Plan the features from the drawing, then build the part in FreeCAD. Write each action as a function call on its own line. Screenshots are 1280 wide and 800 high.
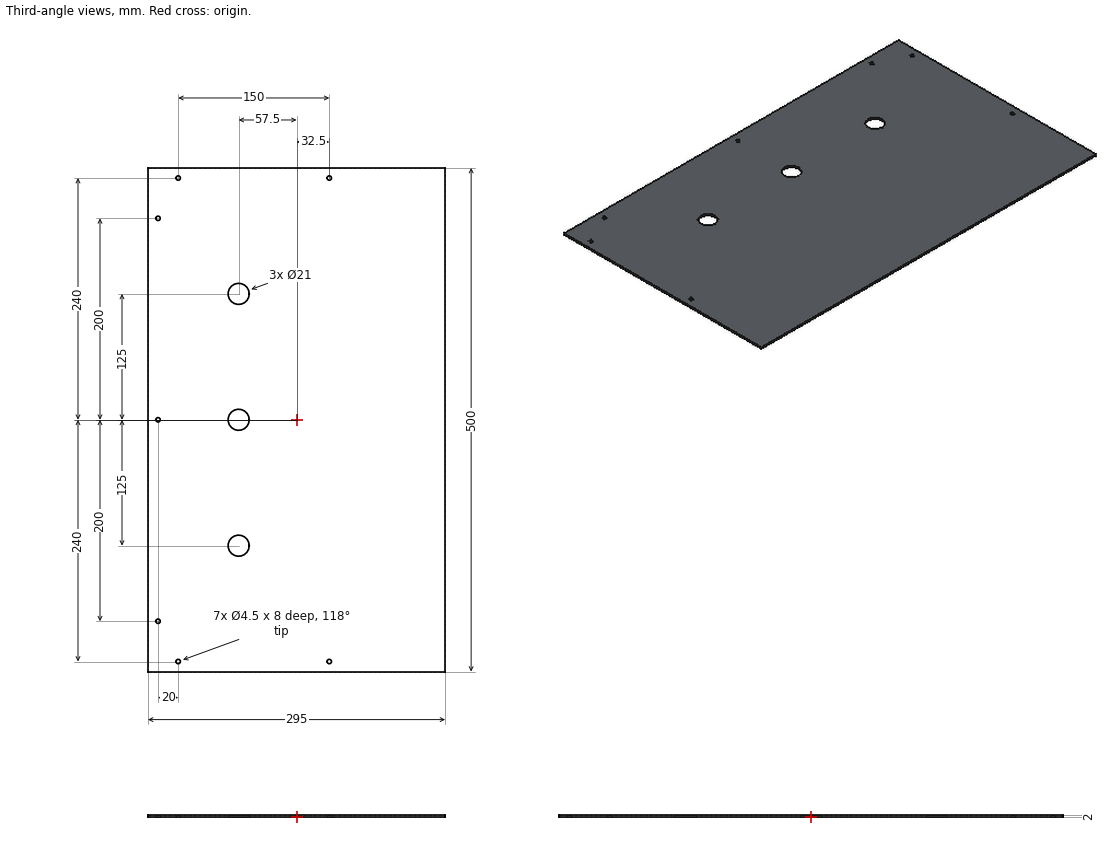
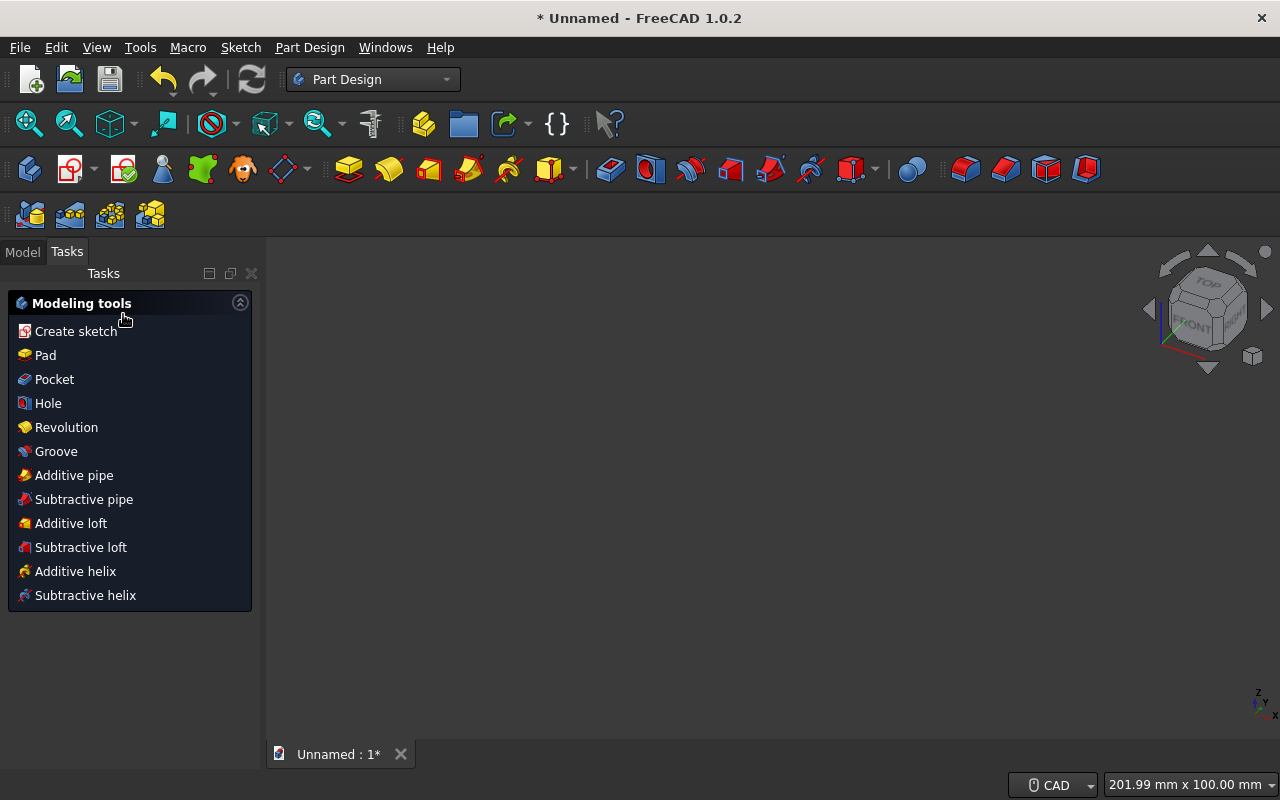
click(350, 170)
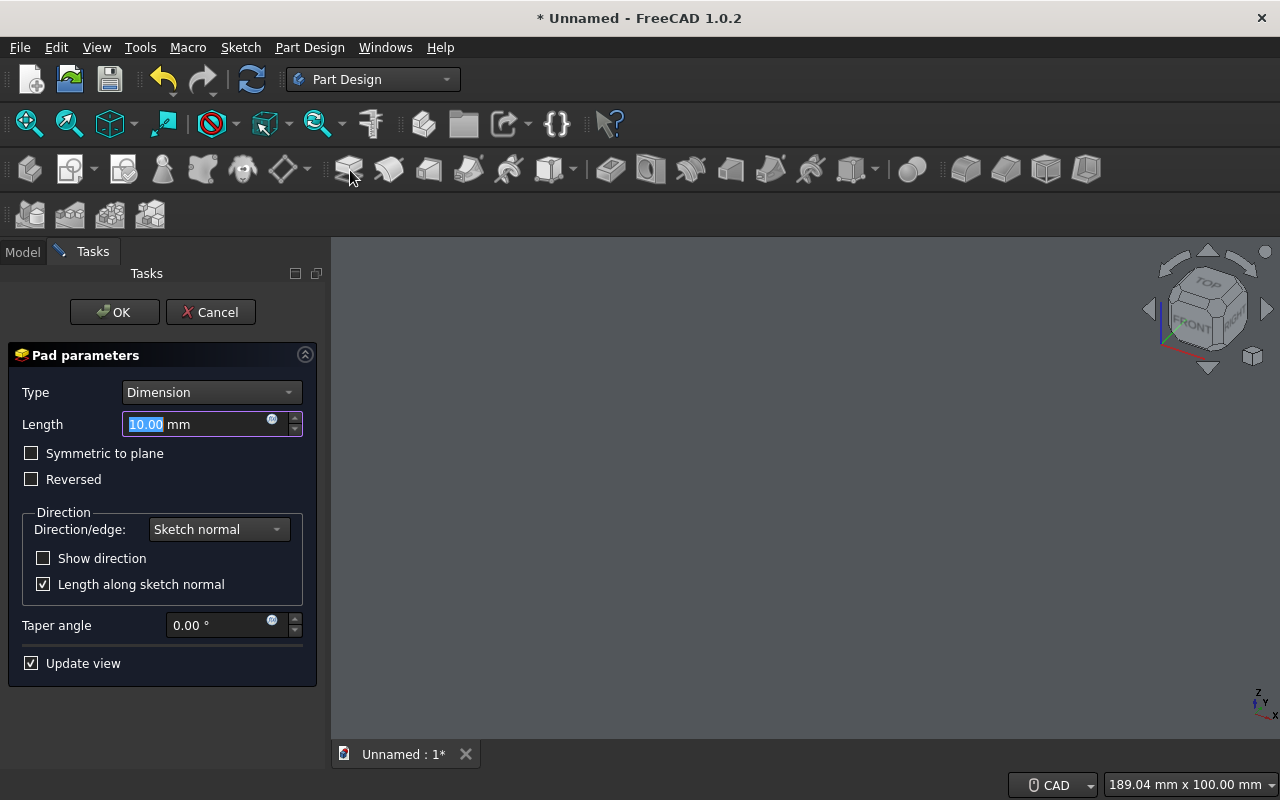
text(2)
key(Tab)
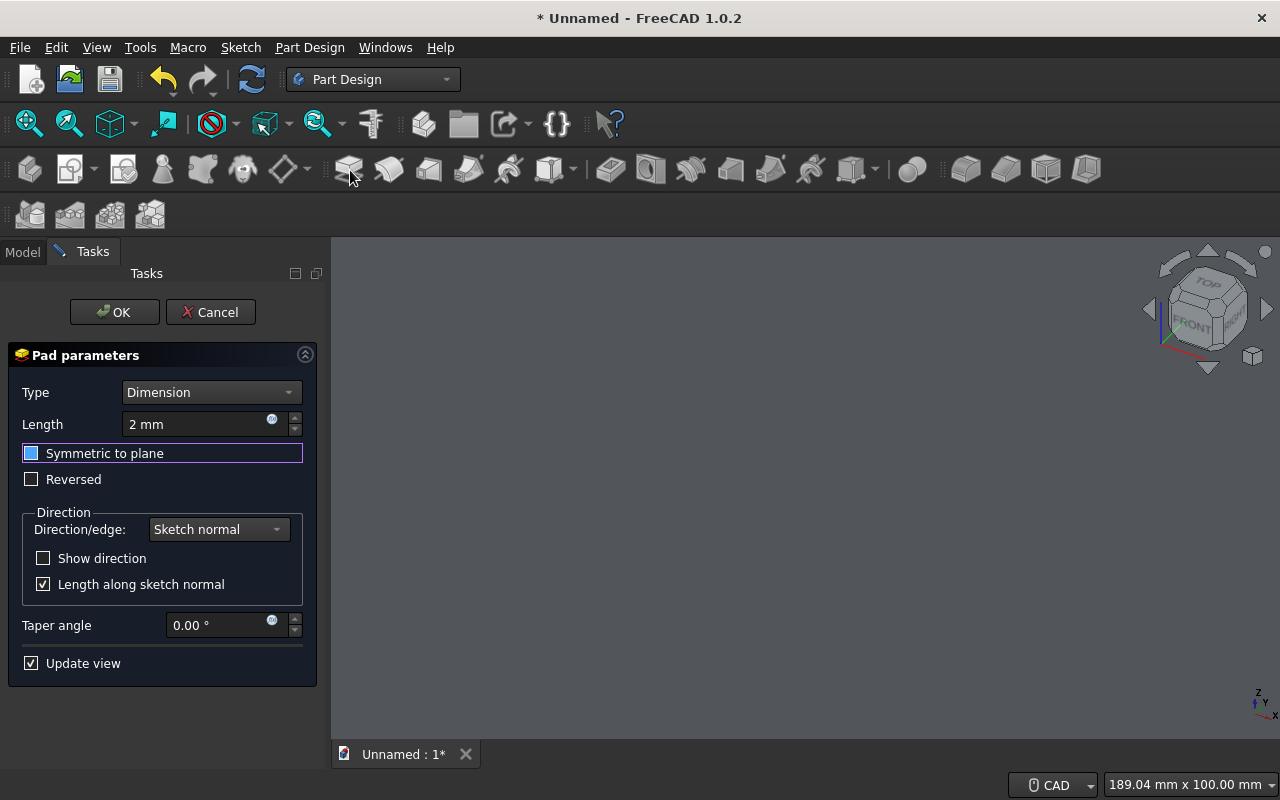
click(115, 312)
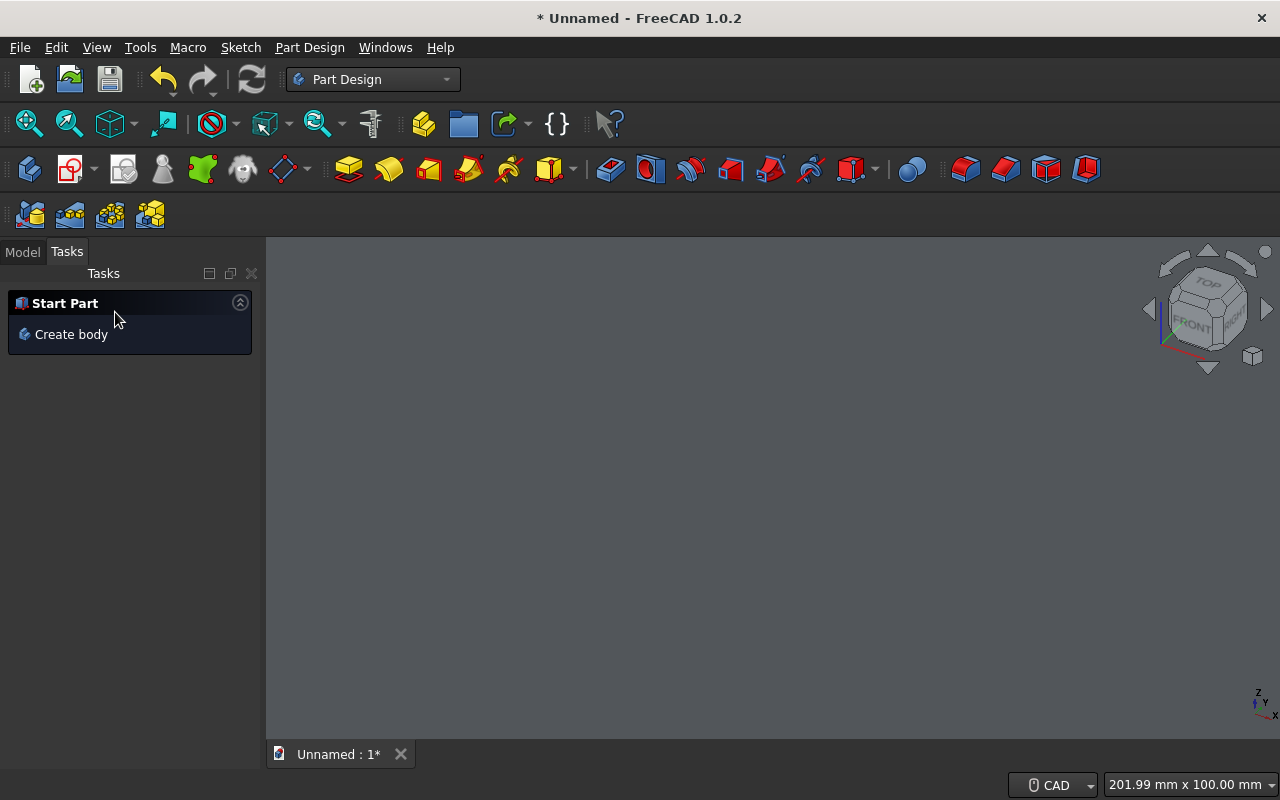
click(30, 124)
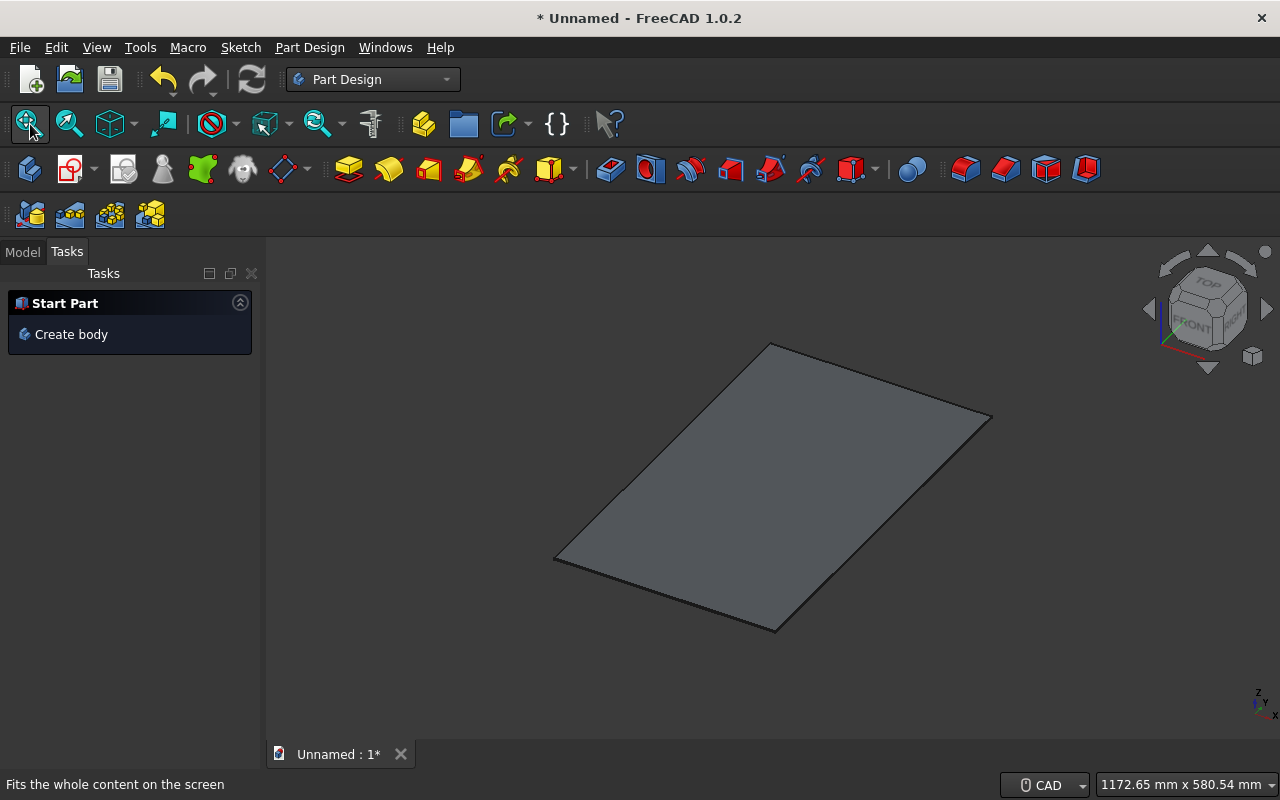
click(804, 456)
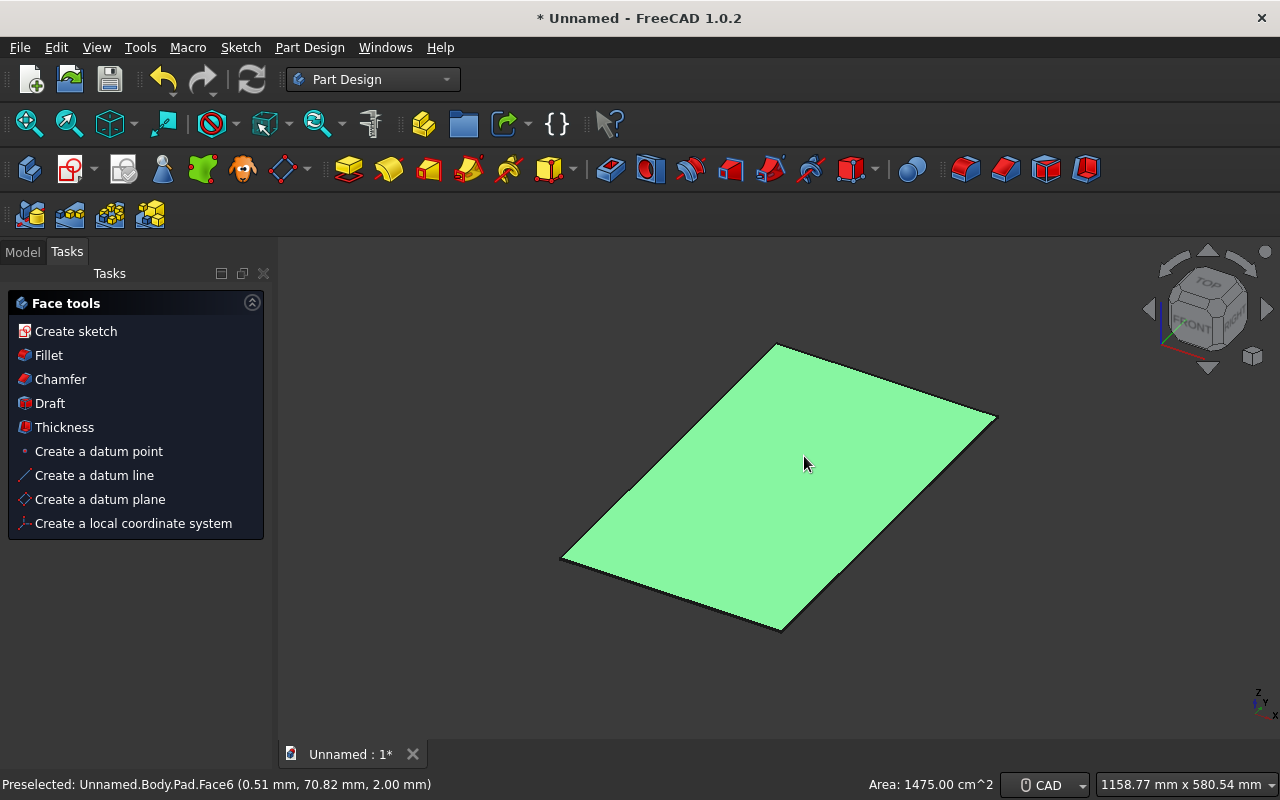
click(70, 170)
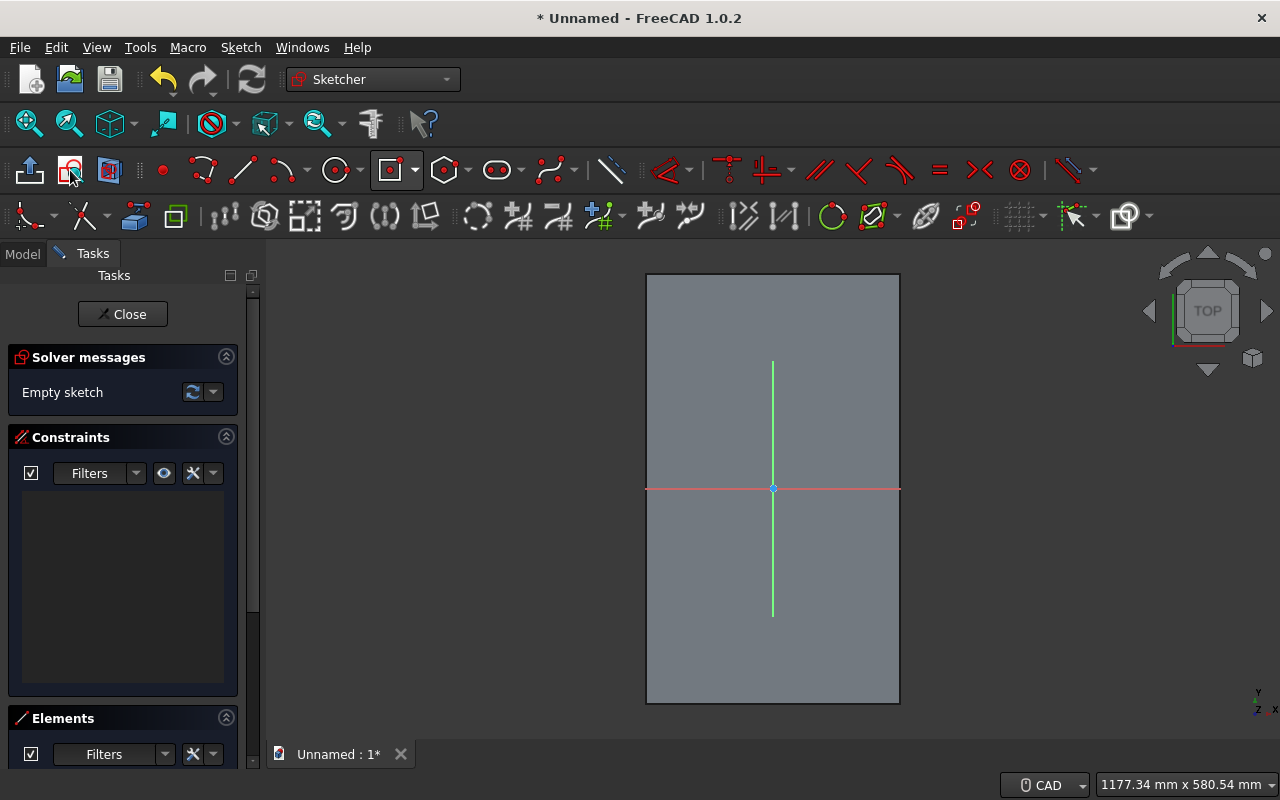
scroll(599, 489, down, 1)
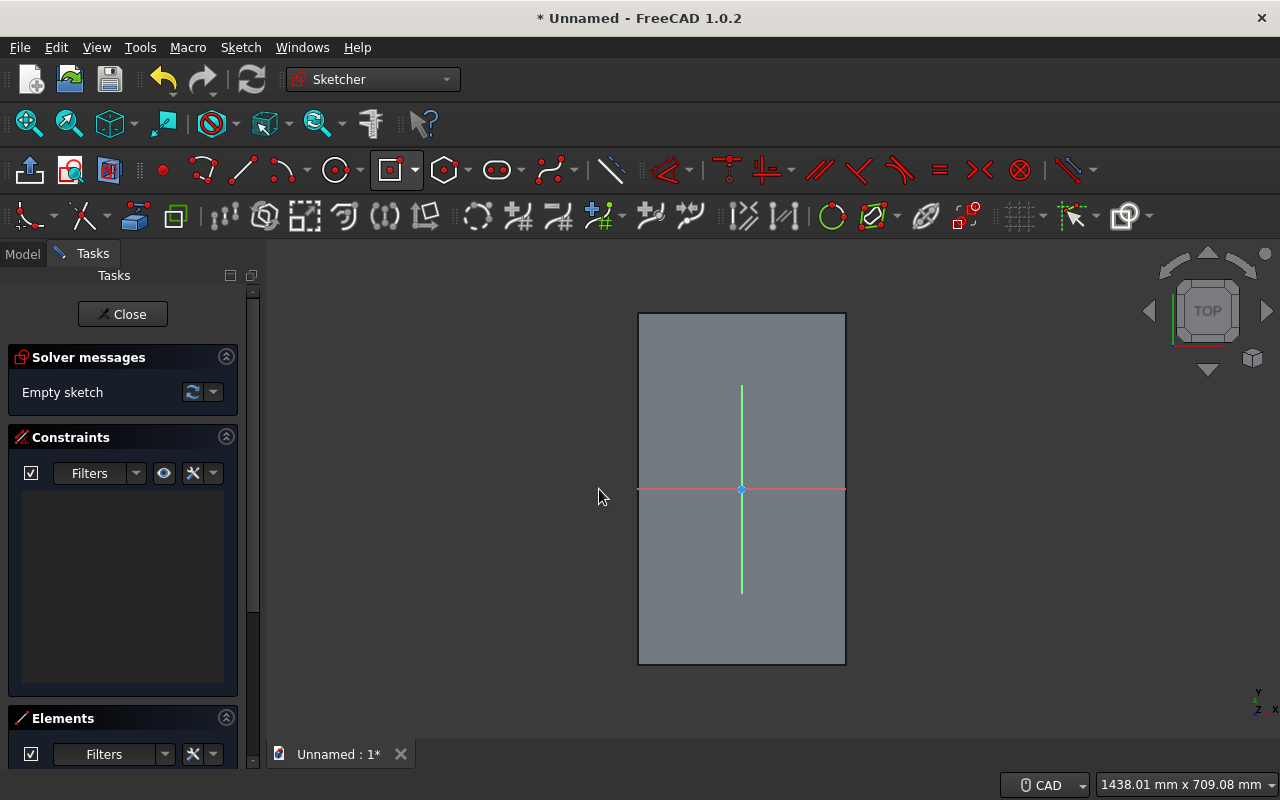
click(336, 170)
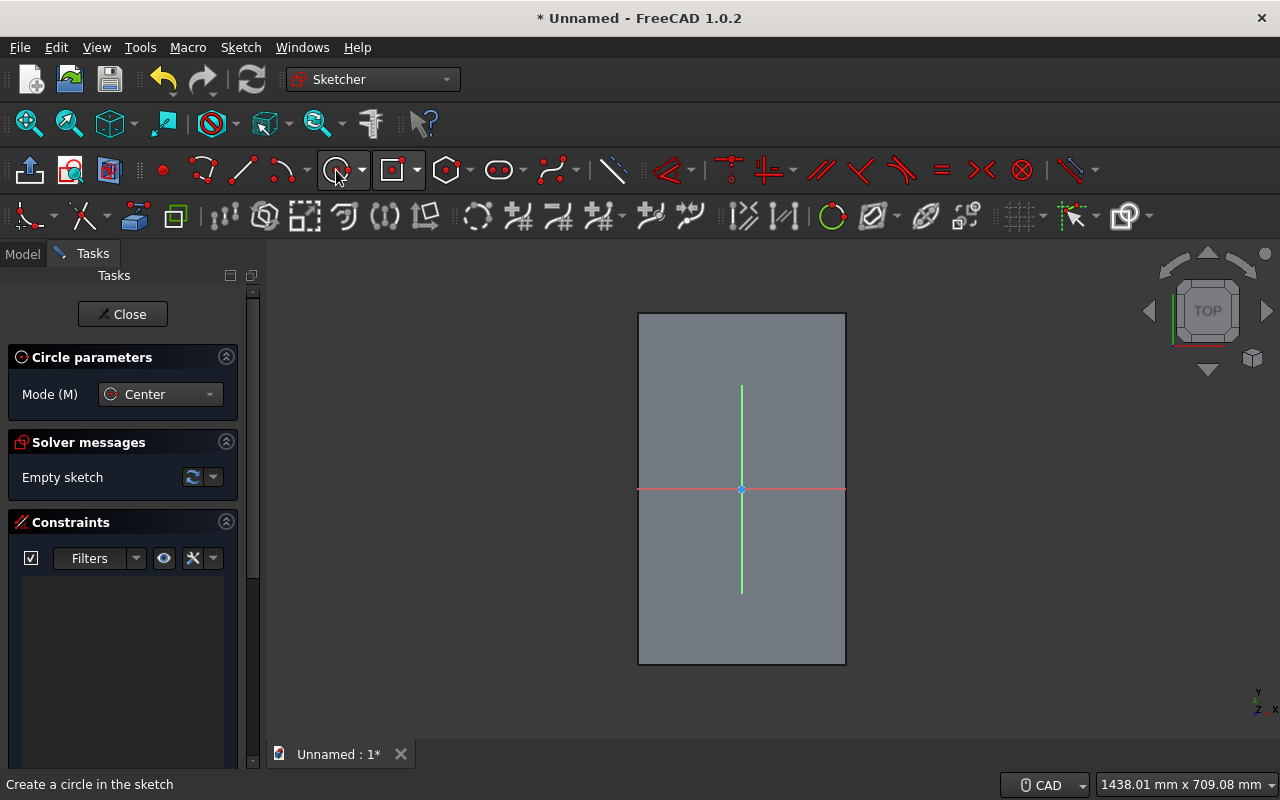
scroll(659, 658, up, 14)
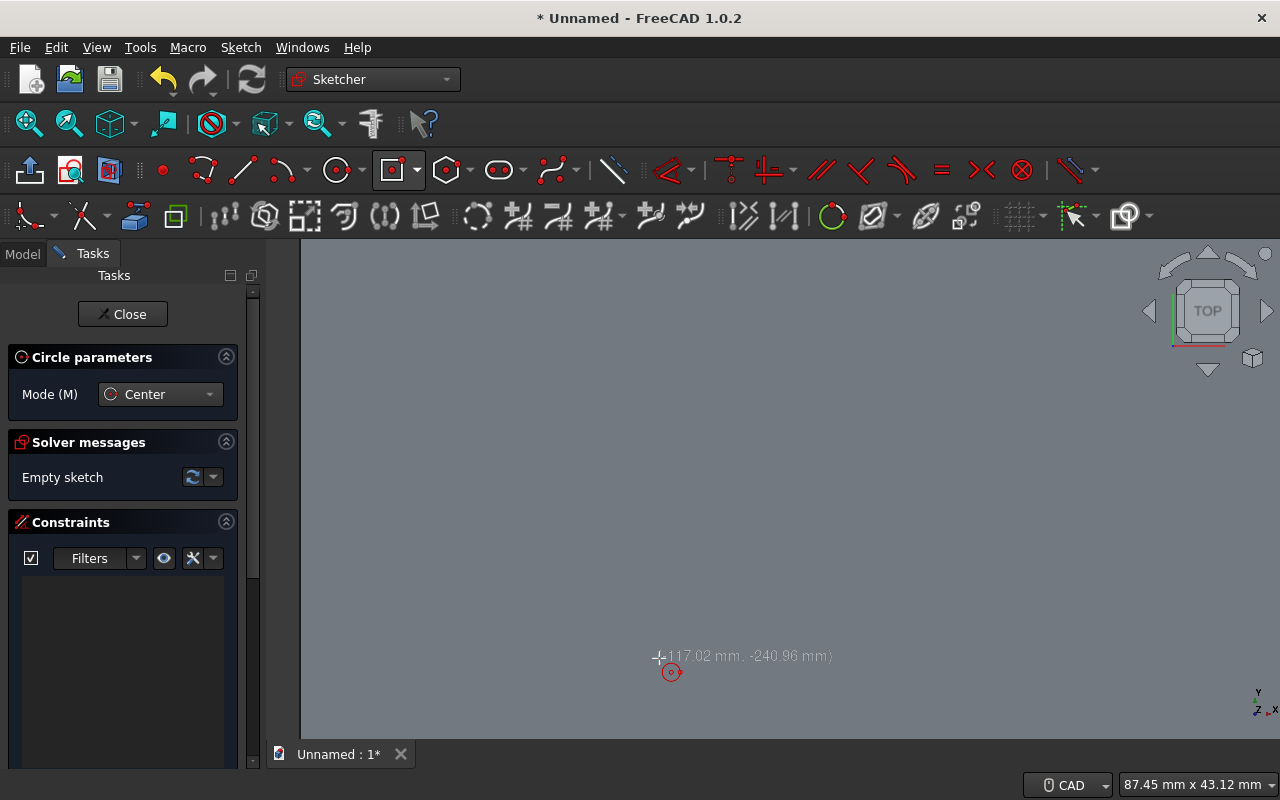
scroll(659, 659, down, 14)